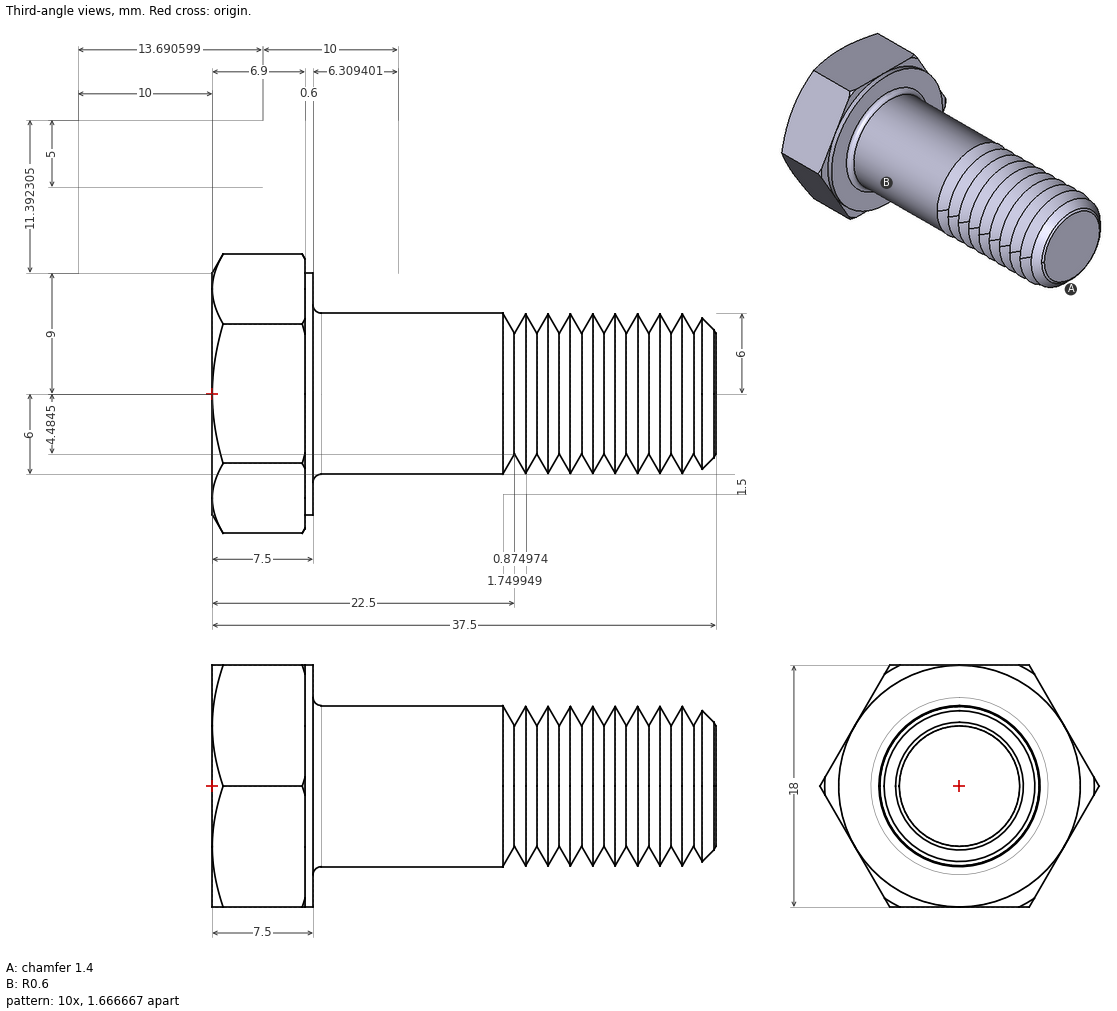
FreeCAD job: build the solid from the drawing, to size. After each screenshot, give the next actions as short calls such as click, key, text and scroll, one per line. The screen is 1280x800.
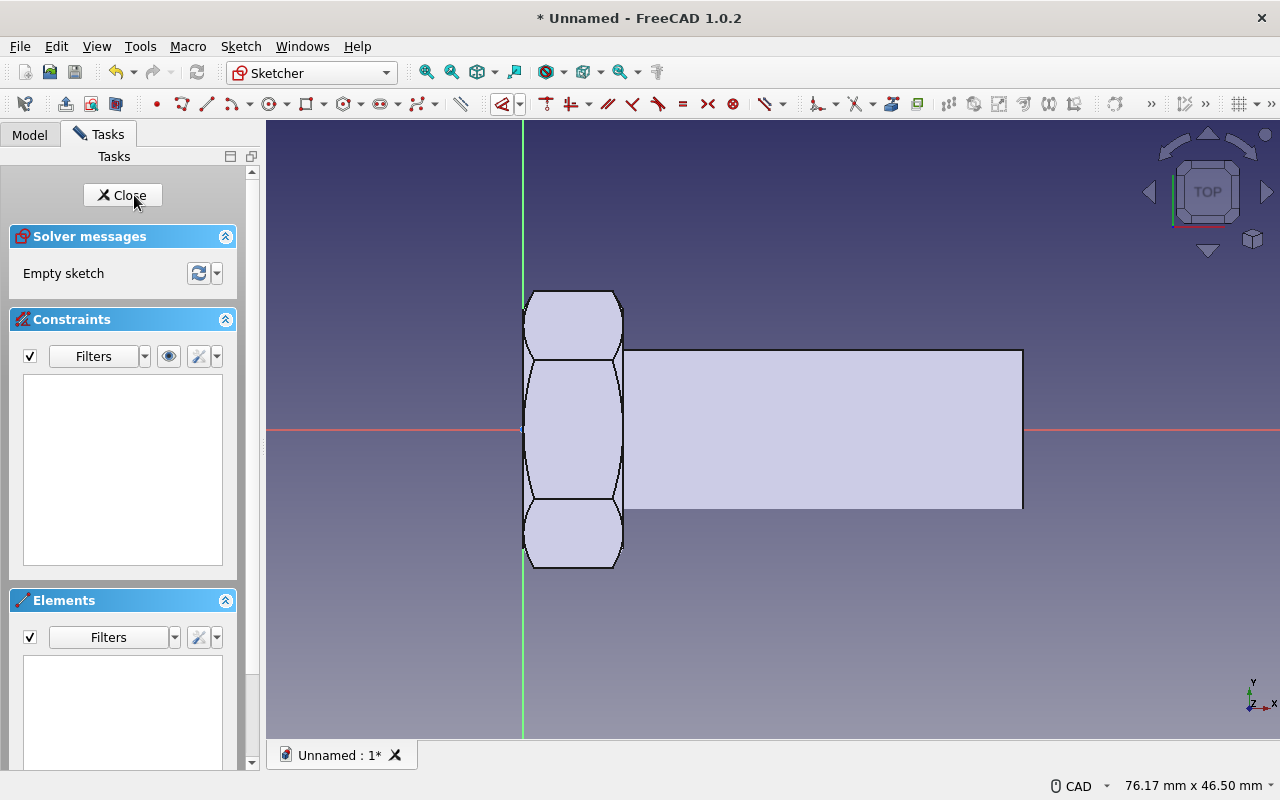
click(116, 104)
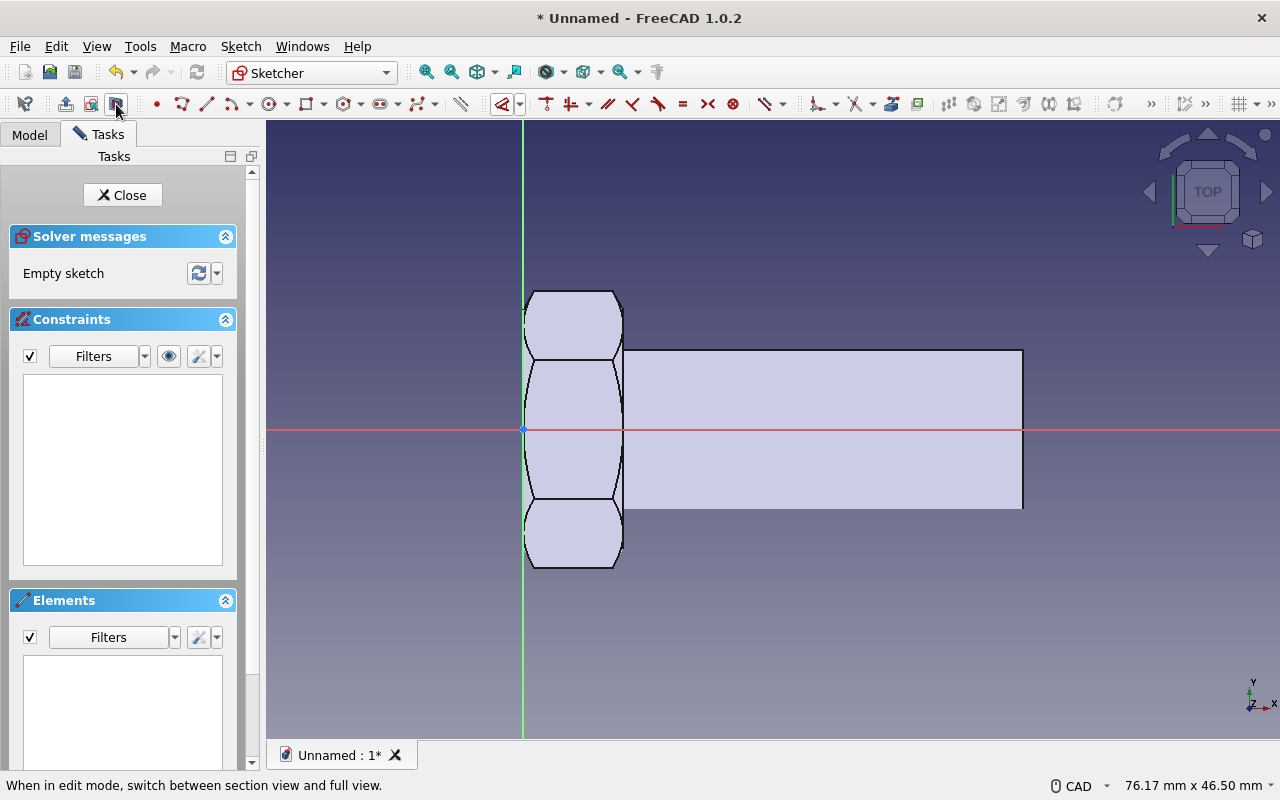
scroll(1115, 711, down, 1)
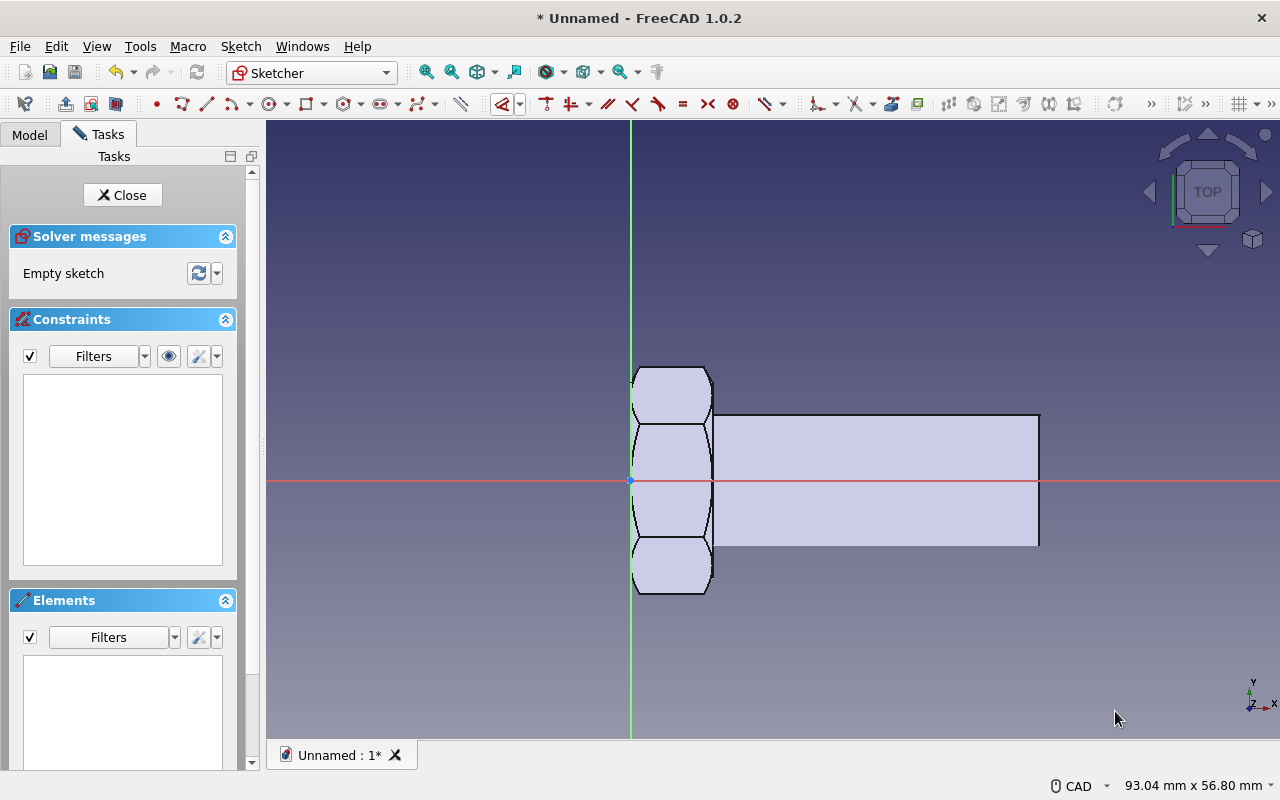
scroll(632, 297, up, 3)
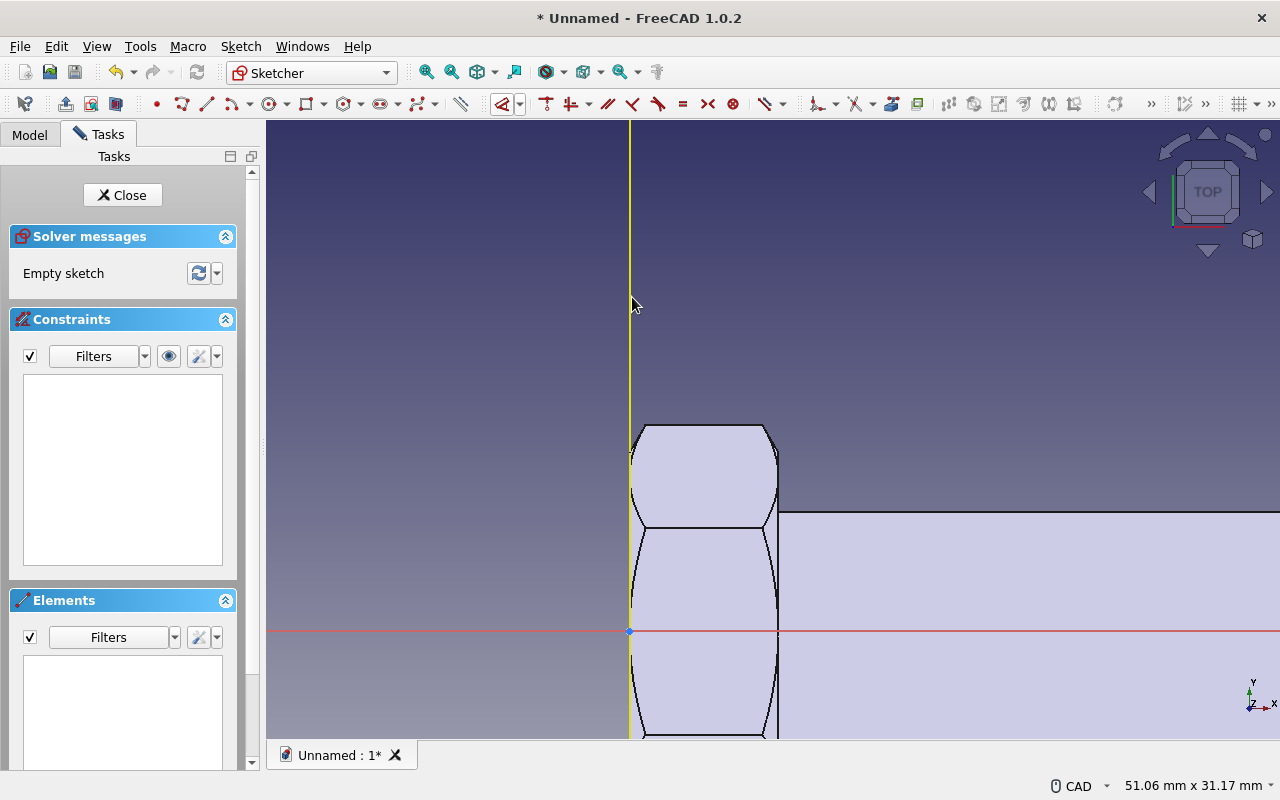
click(306, 104)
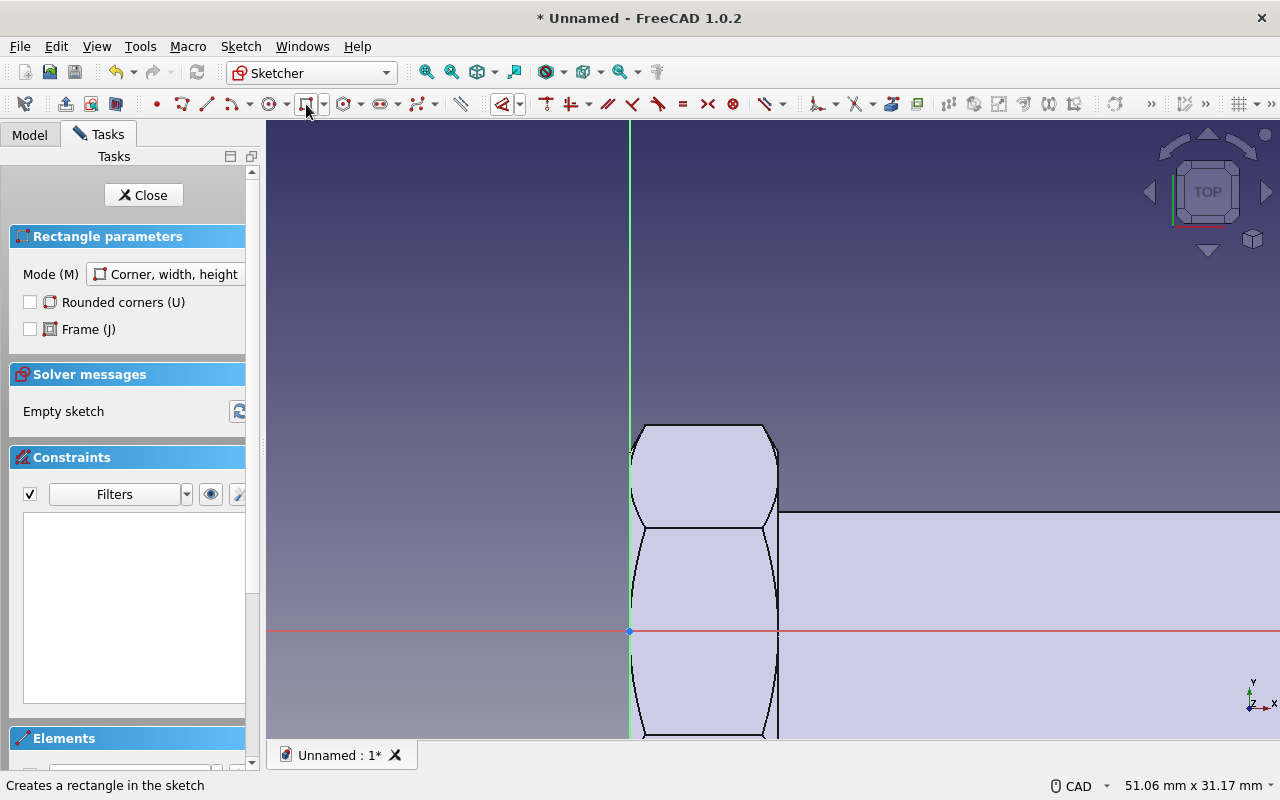
scroll(767, 227, up, 2)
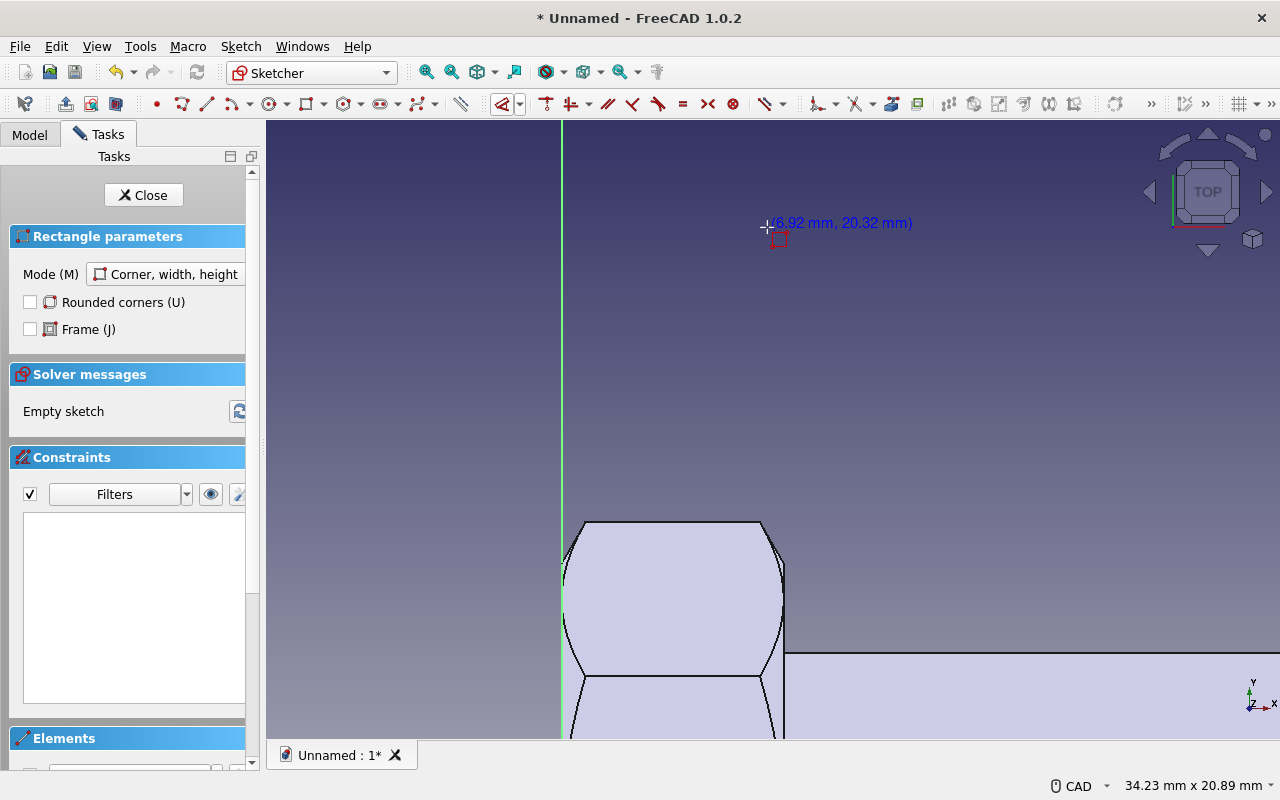
click(766, 226)
click(784, 564)
key(Escape)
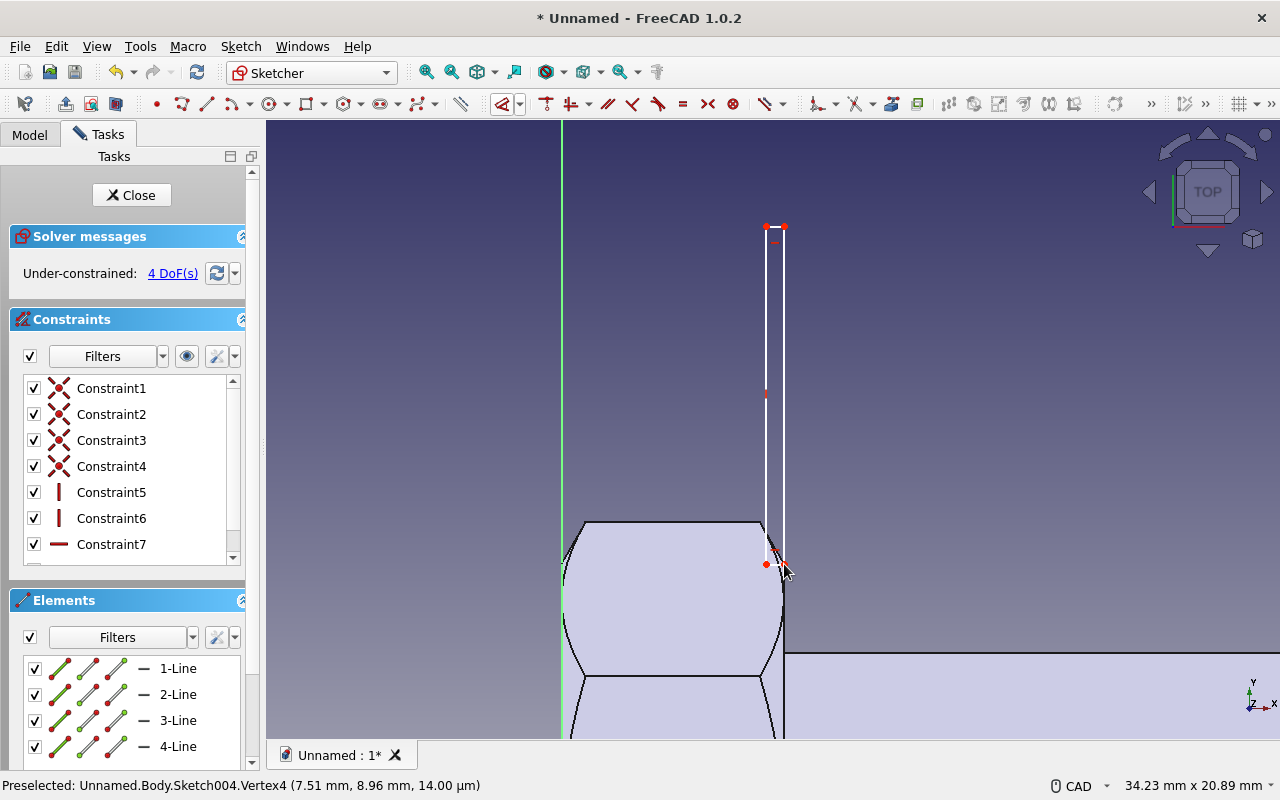
click(766, 565)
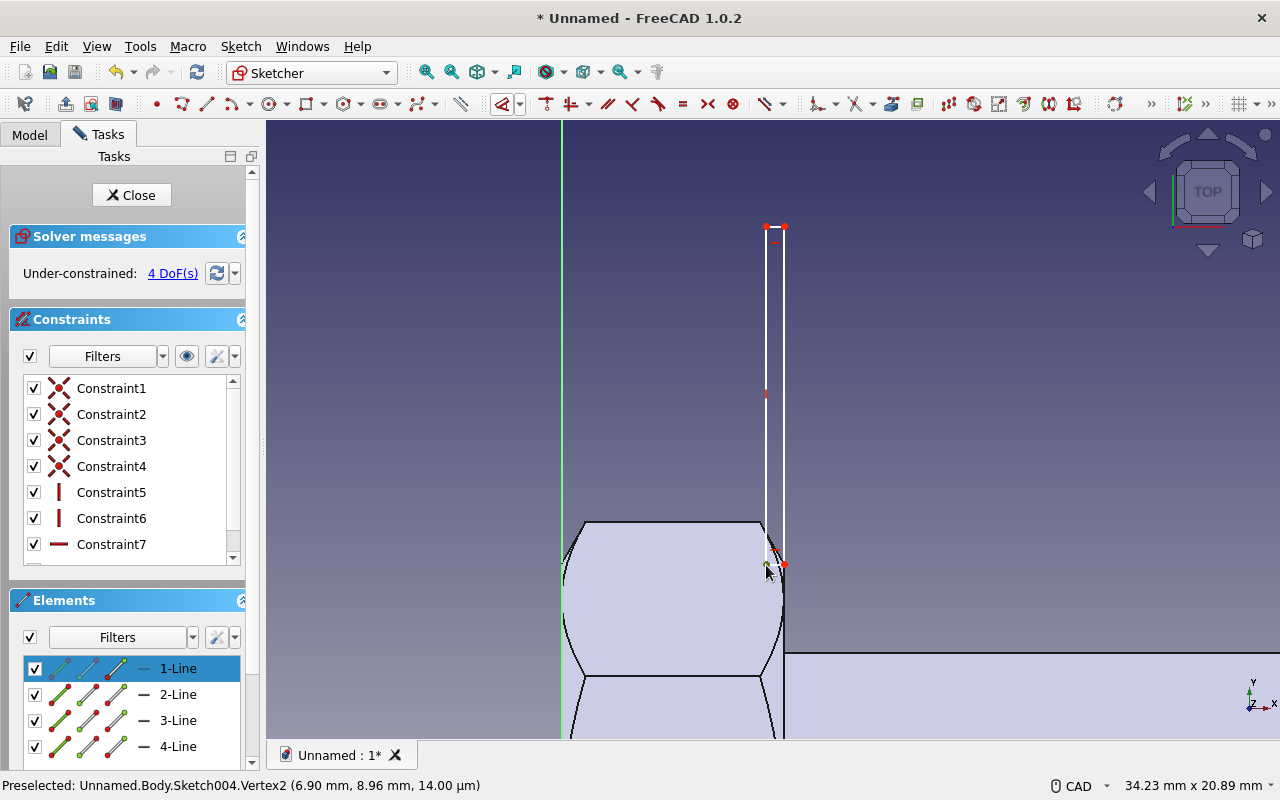
click(520, 104)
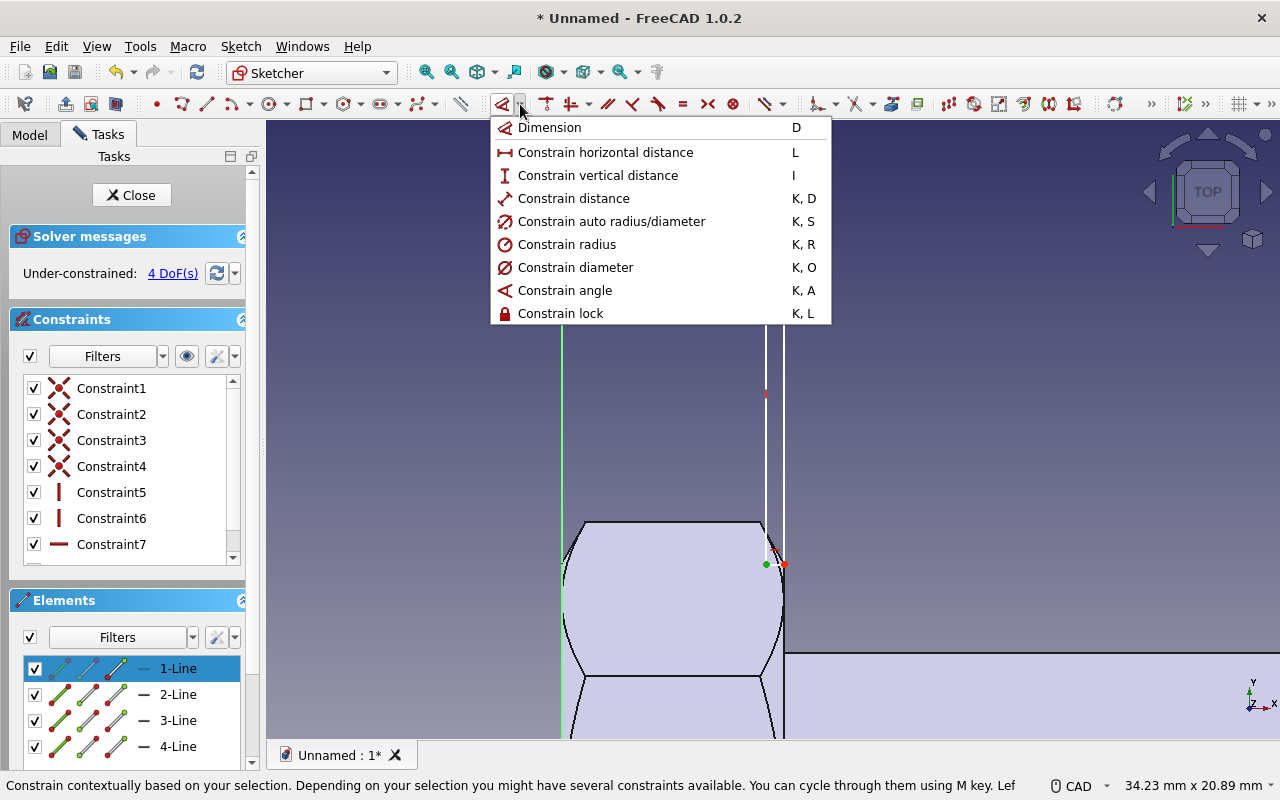
click(661, 176)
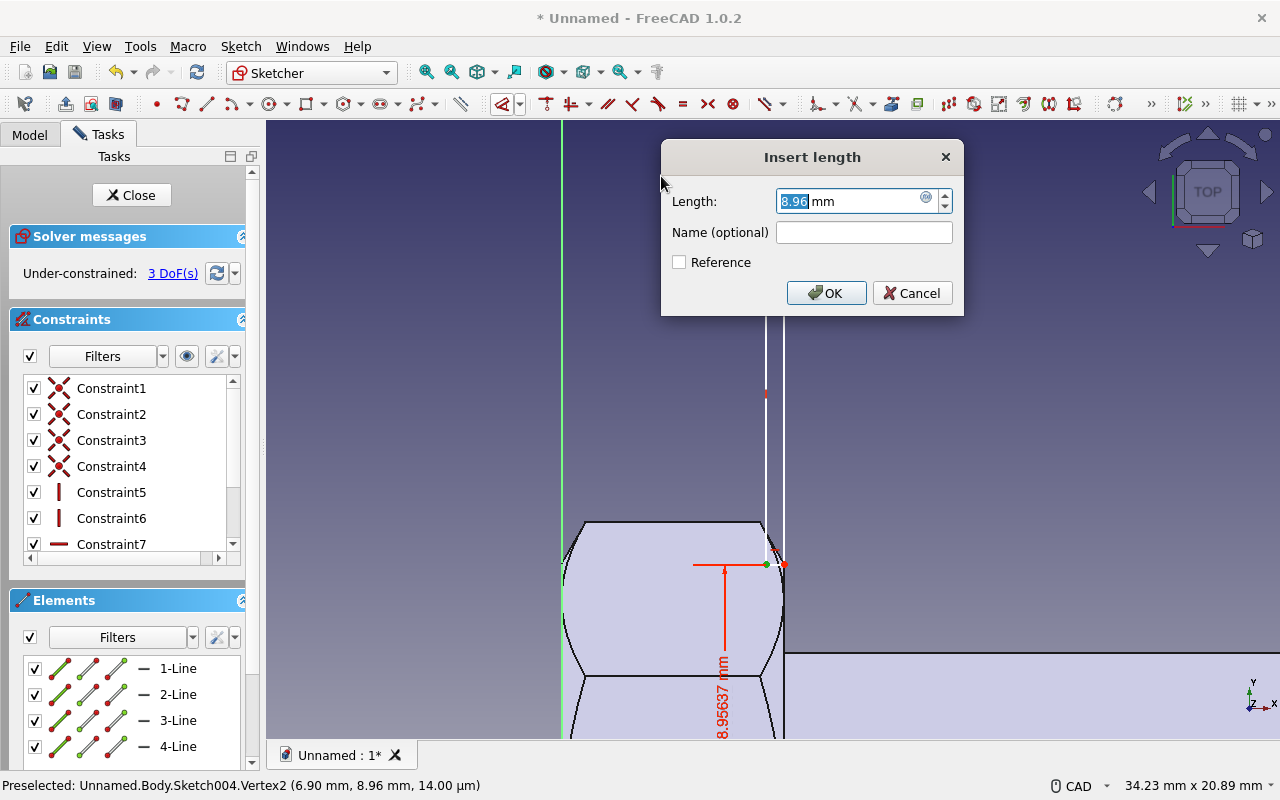
text(9)
key(Return)